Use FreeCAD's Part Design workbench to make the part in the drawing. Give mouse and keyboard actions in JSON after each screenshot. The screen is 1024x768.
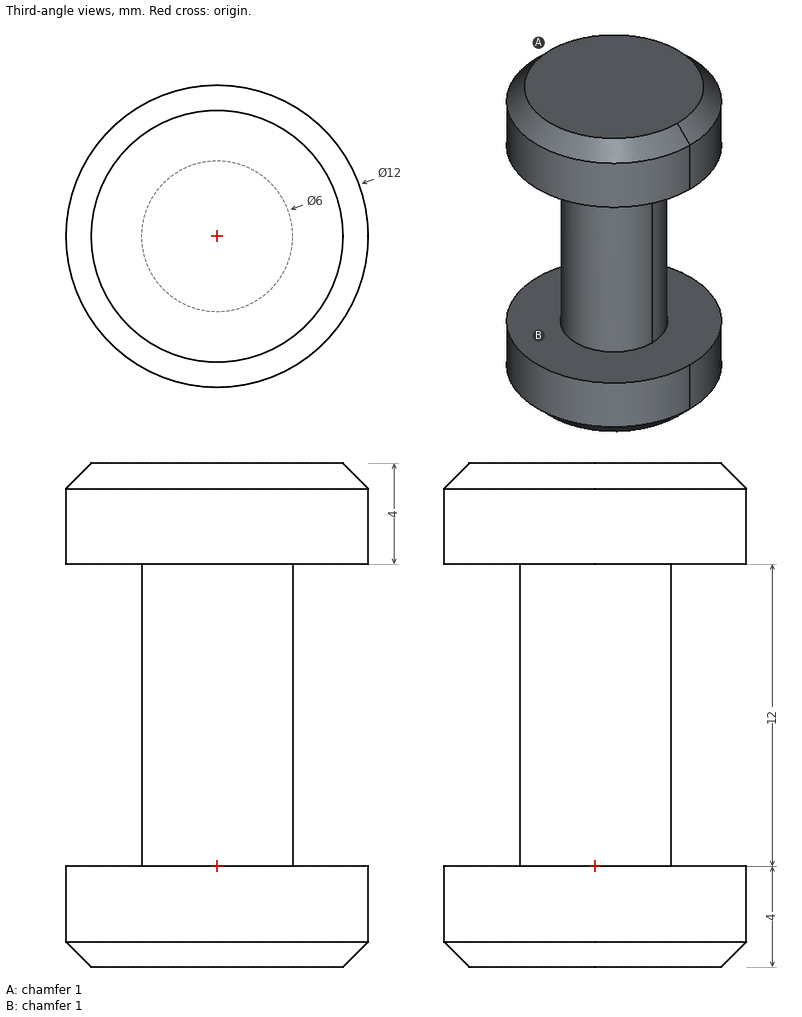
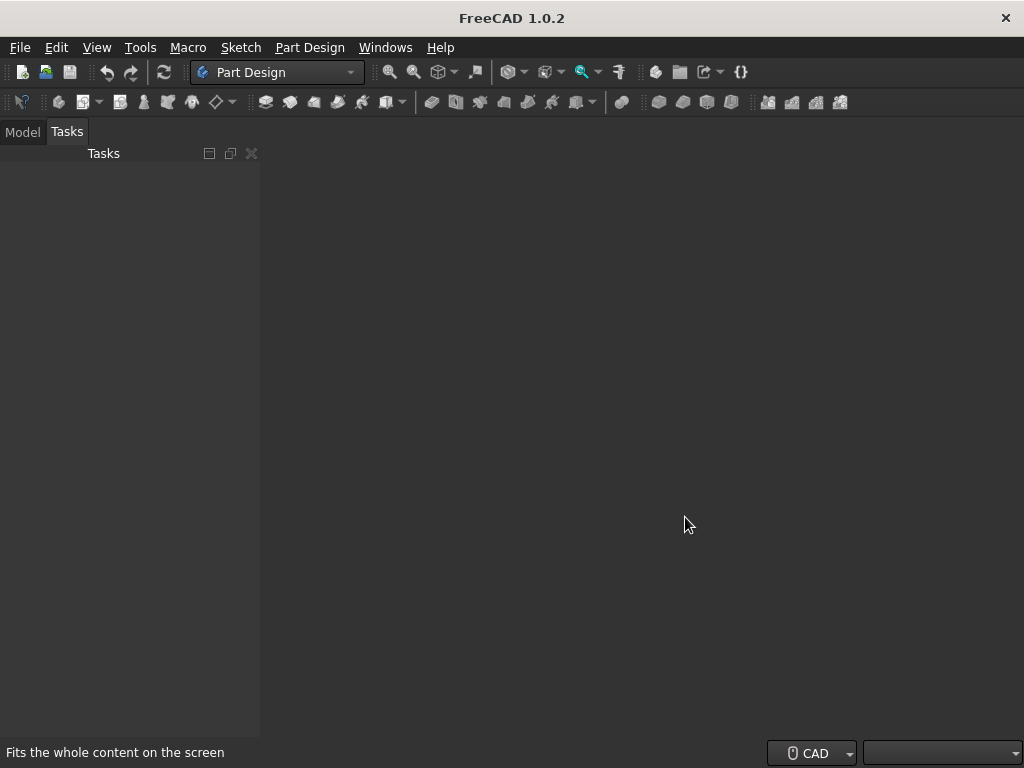
{"action": "left_click", "coordinate": [22, 72]}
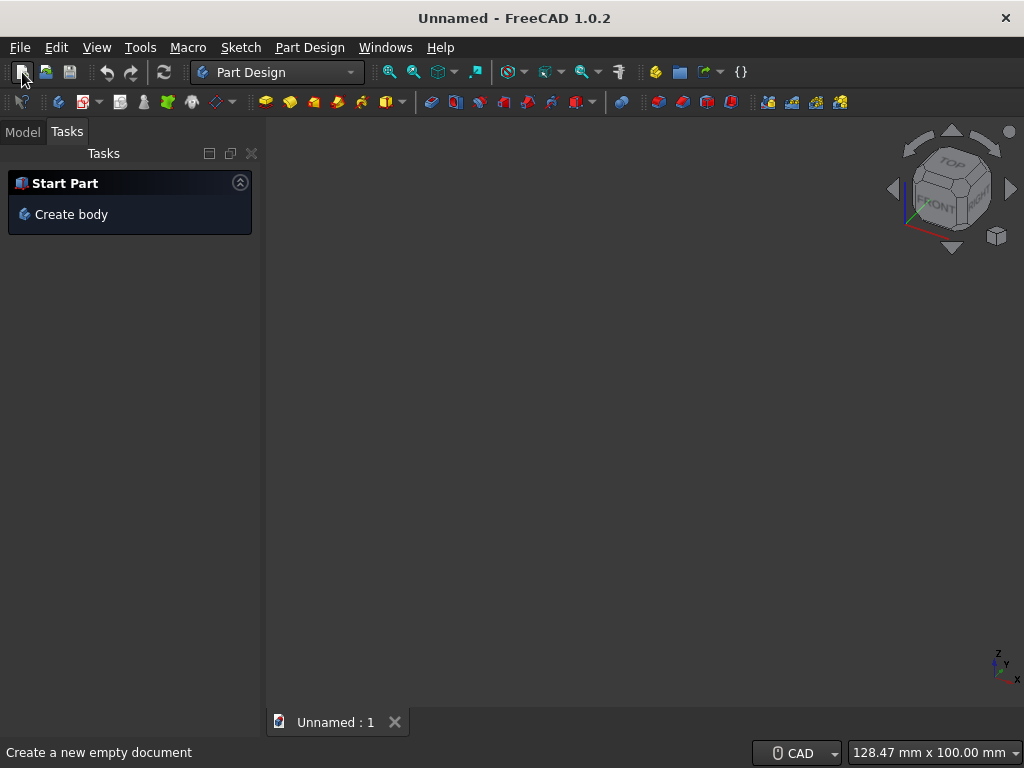
{"action": "left_click", "coordinate": [84, 102]}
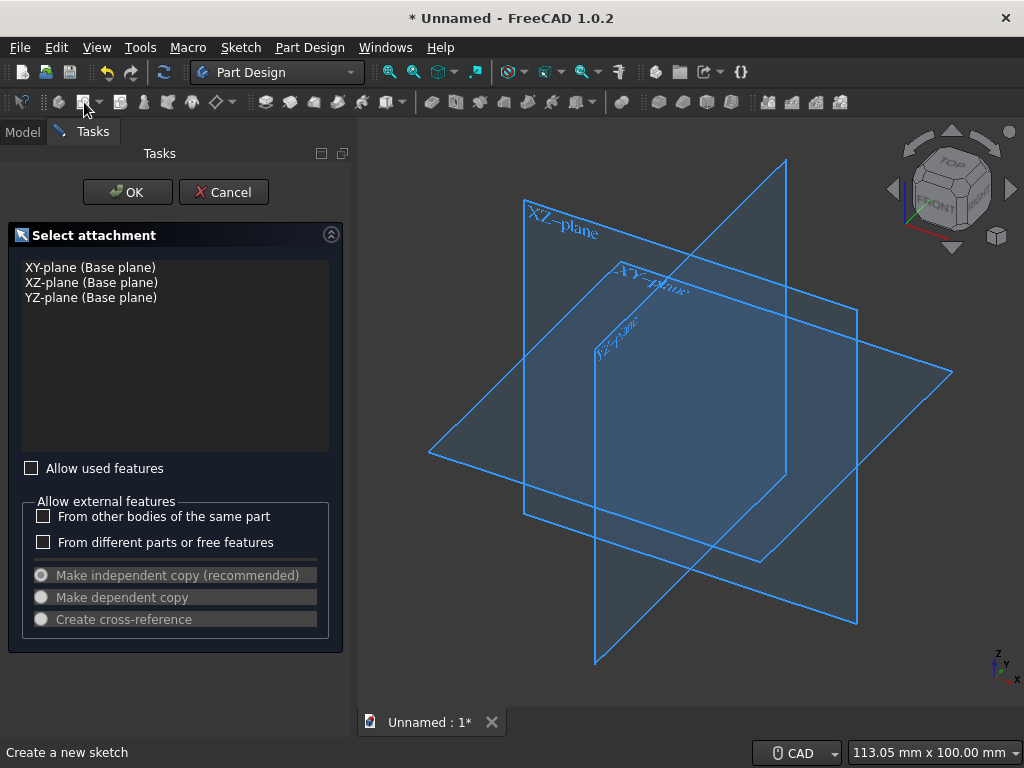
{"action": "left_click", "coordinate": [82, 268]}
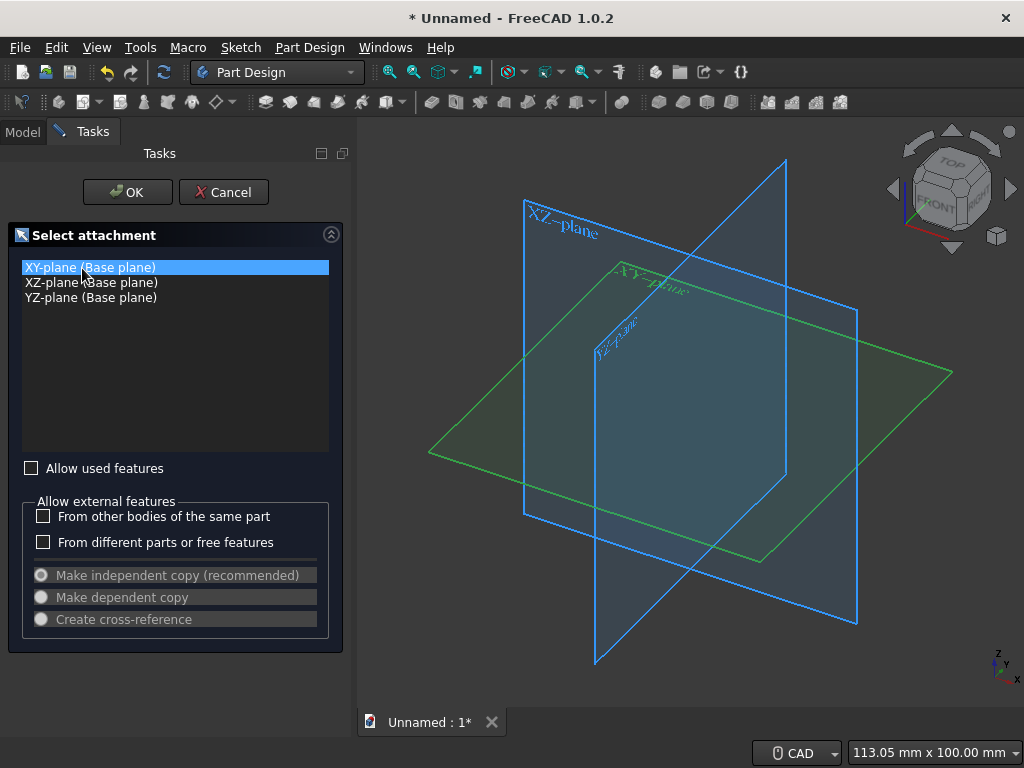
{"action": "left_click", "coordinate": [128, 192]}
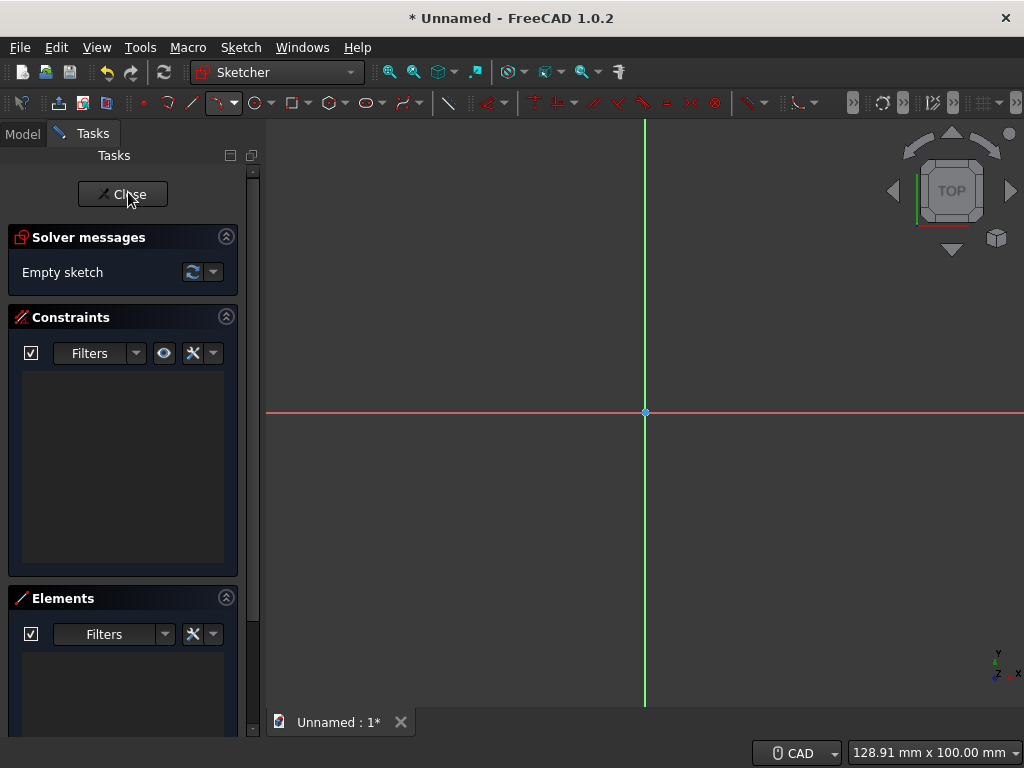
{"action": "scroll", "coordinate": [652, 413], "scroll_direction": "up", "scroll_amount": 12}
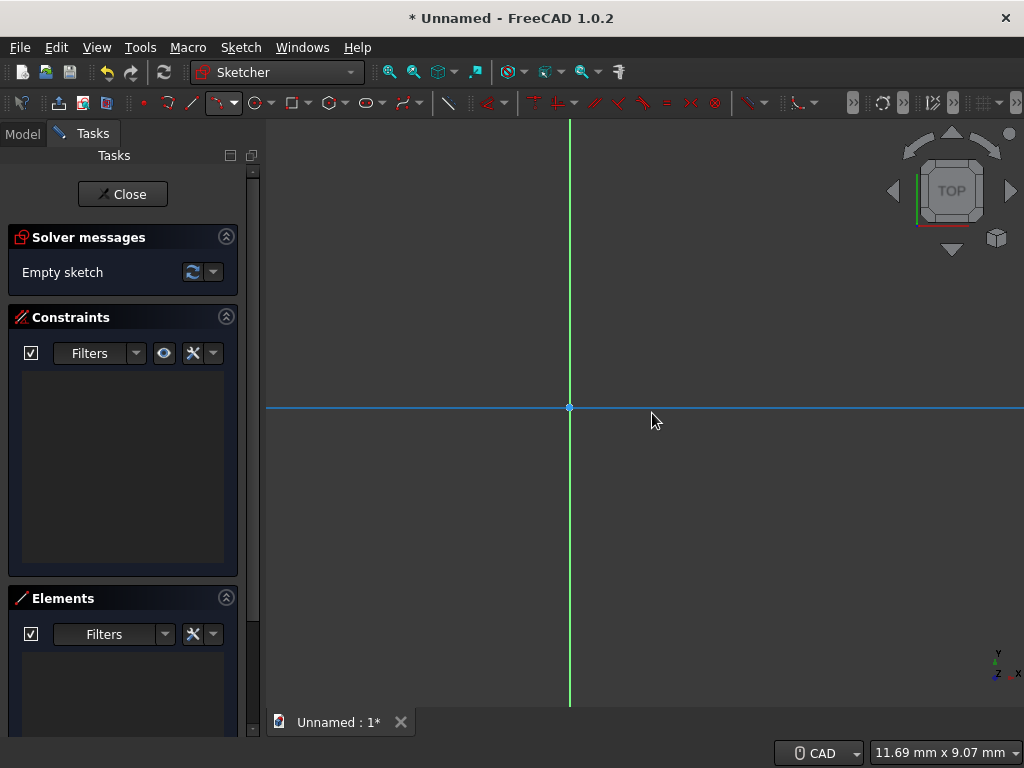
{"action": "key", "text": "g c"}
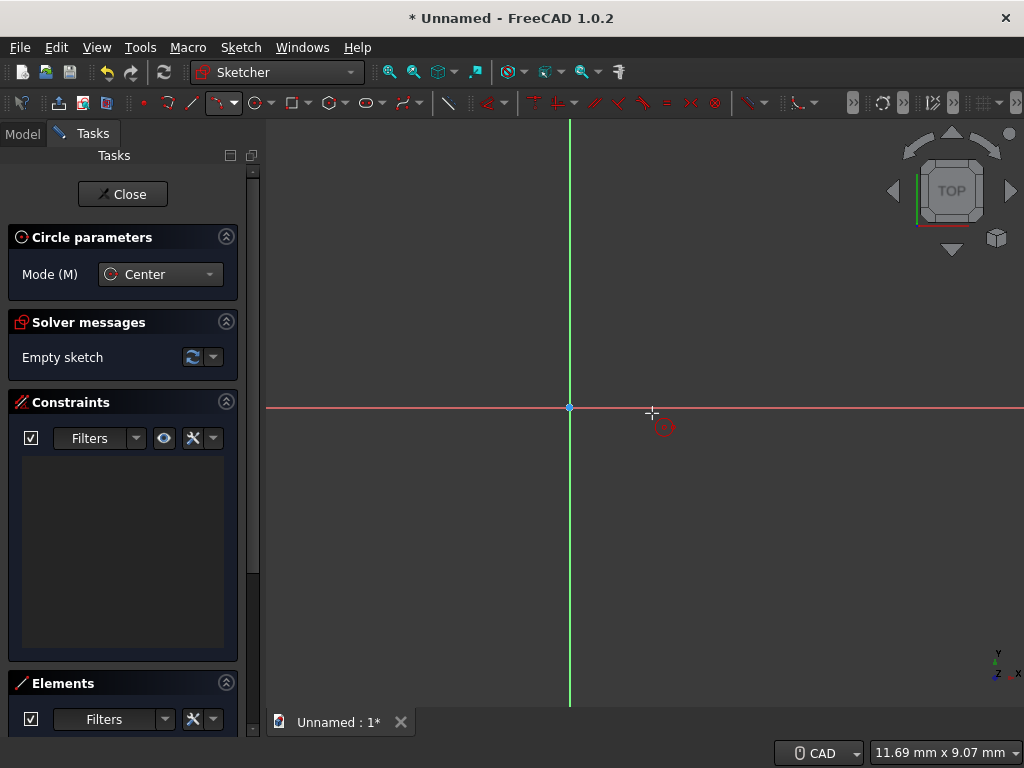
{"action": "left_click", "coordinate": [570, 408]}
{"action": "left_click", "coordinate": [707, 270]}
{"action": "key", "text": "Escape"}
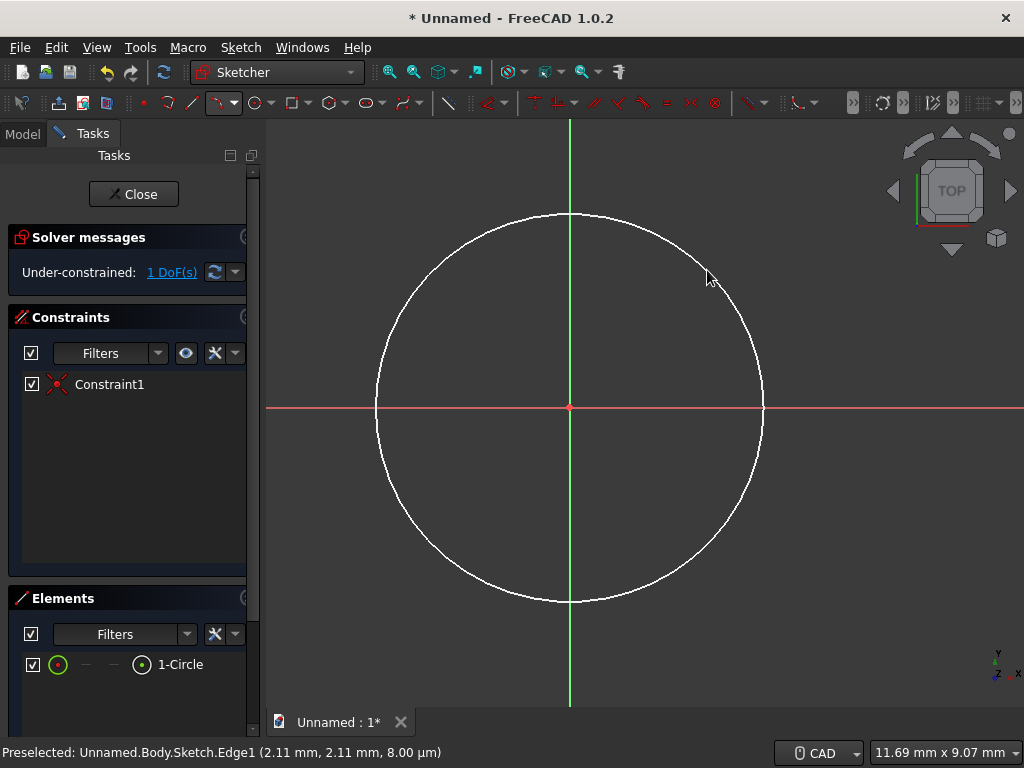
{"action": "left_click", "coordinate": [488, 104]}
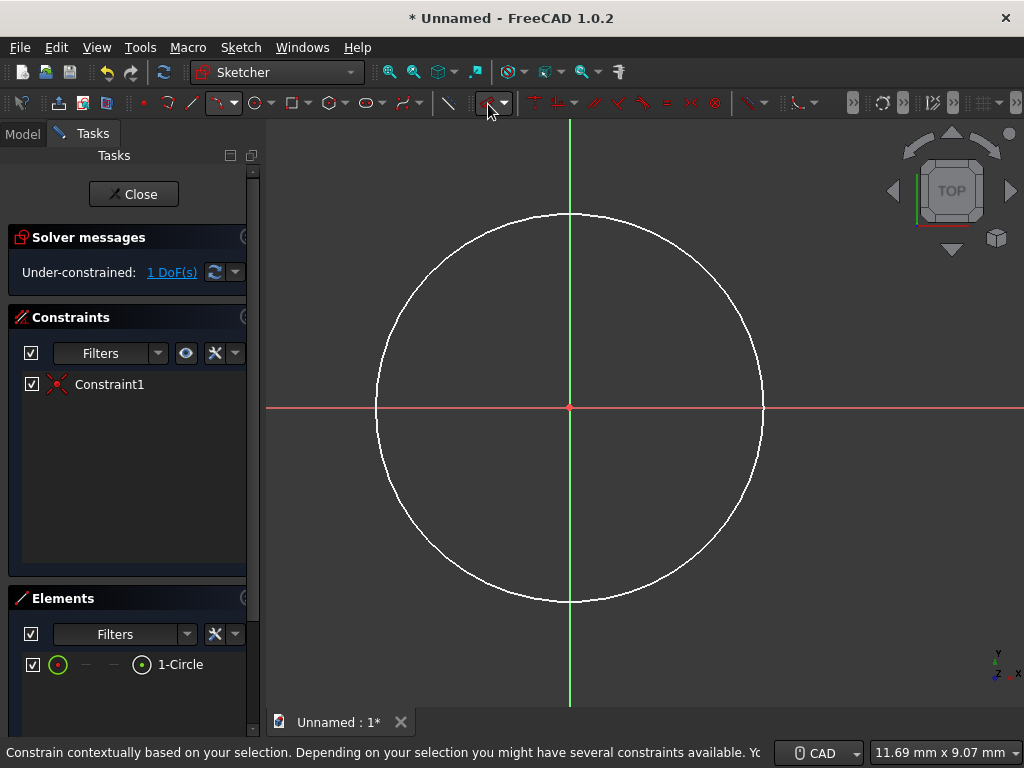
{"action": "left_click", "coordinate": [706, 270]}
{"action": "left_click", "coordinate": [728, 247]}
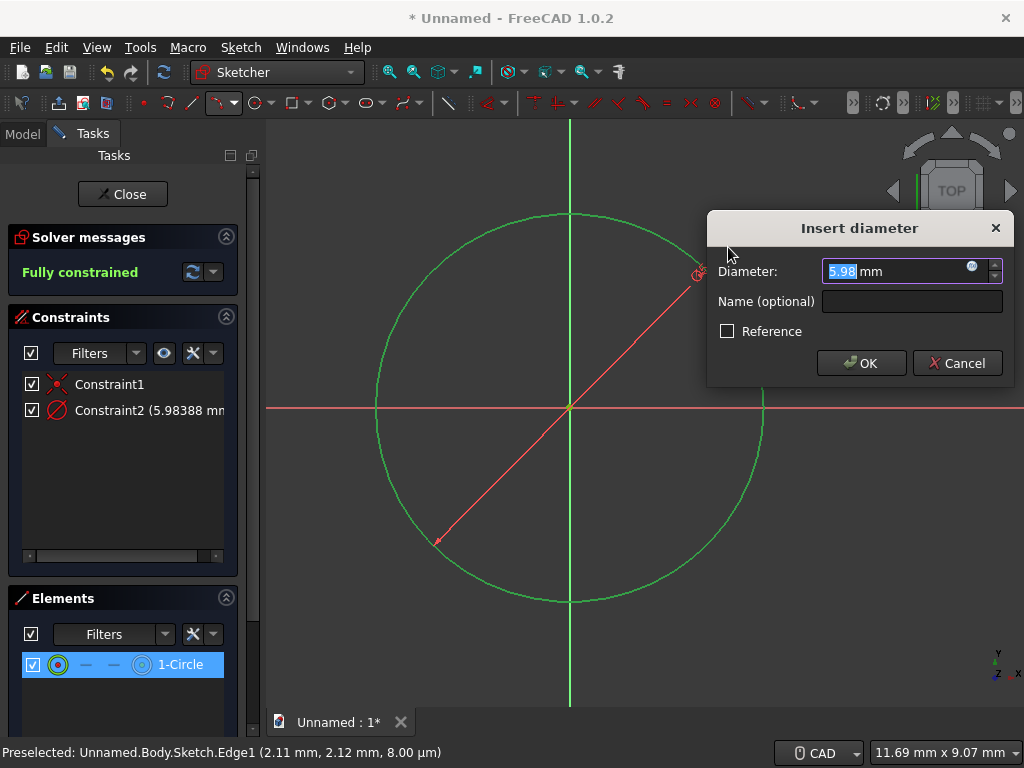
{"action": "type", "text": "6"}
{"action": "key", "text": "Return"}
{"action": "key", "text": "Escape"}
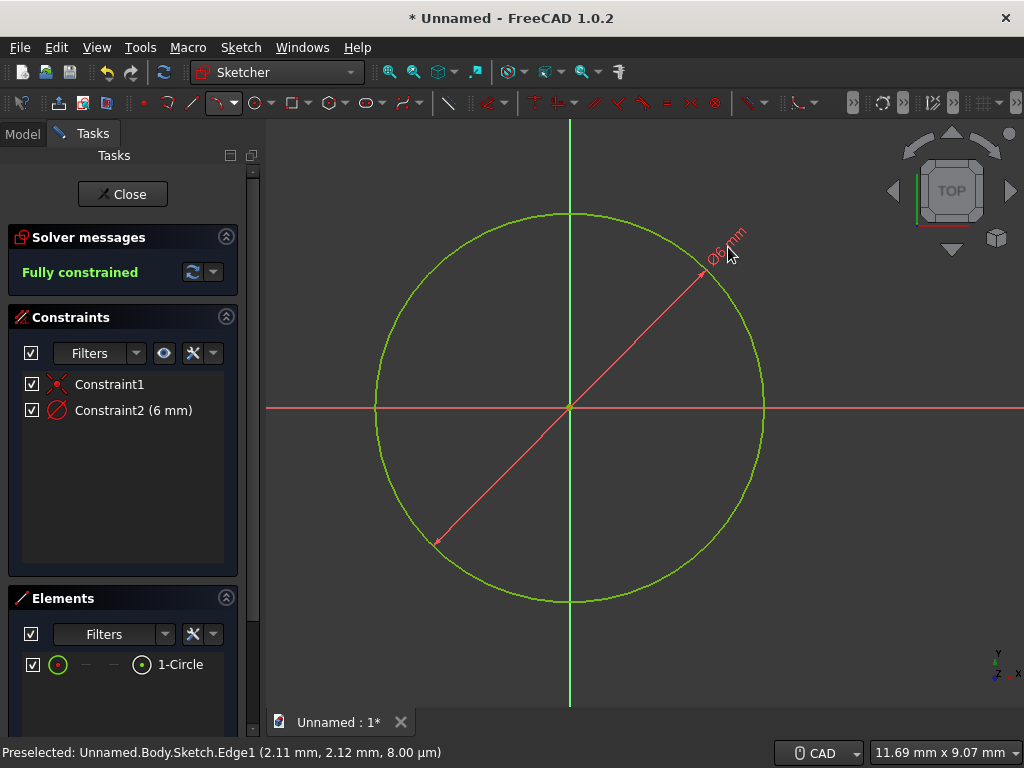
{"action": "left_click", "coordinate": [123, 194]}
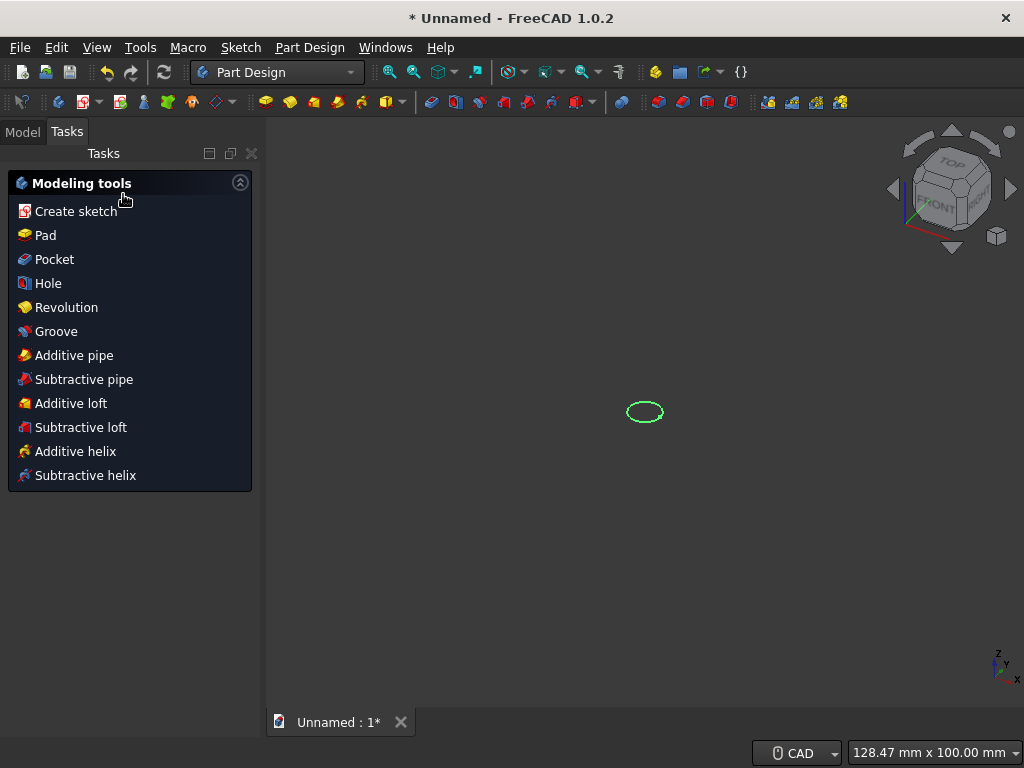
{"action": "left_click", "coordinate": [266, 102]}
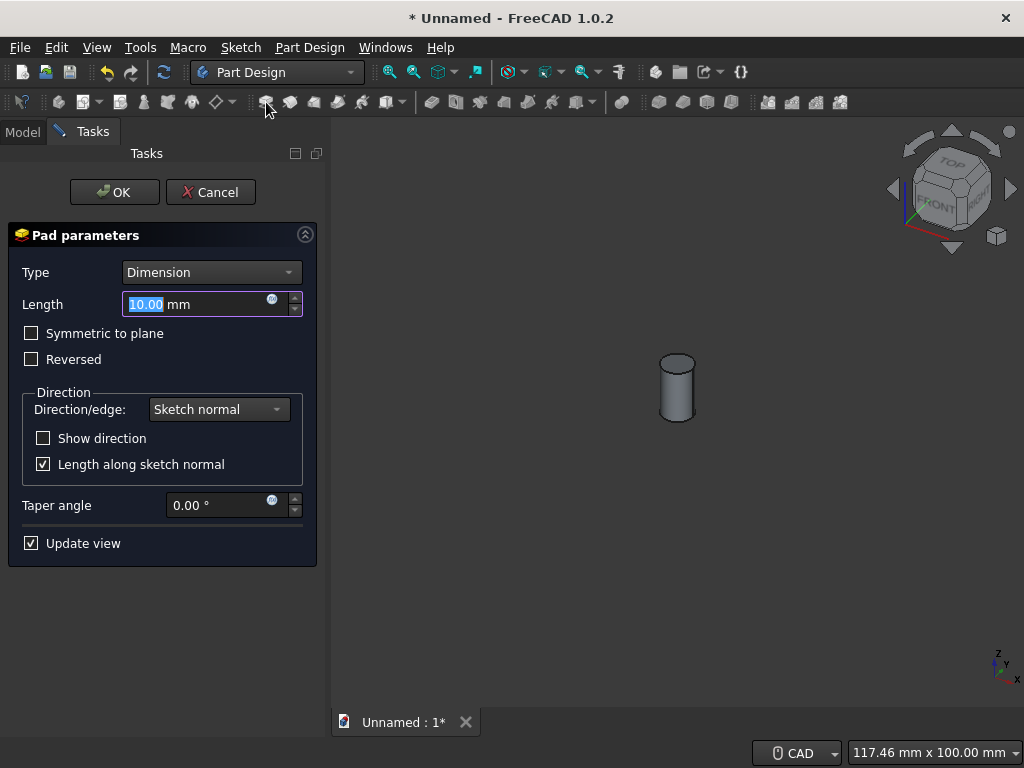
{"action": "type", "text": "12"}
{"action": "key", "text": "Tab"}